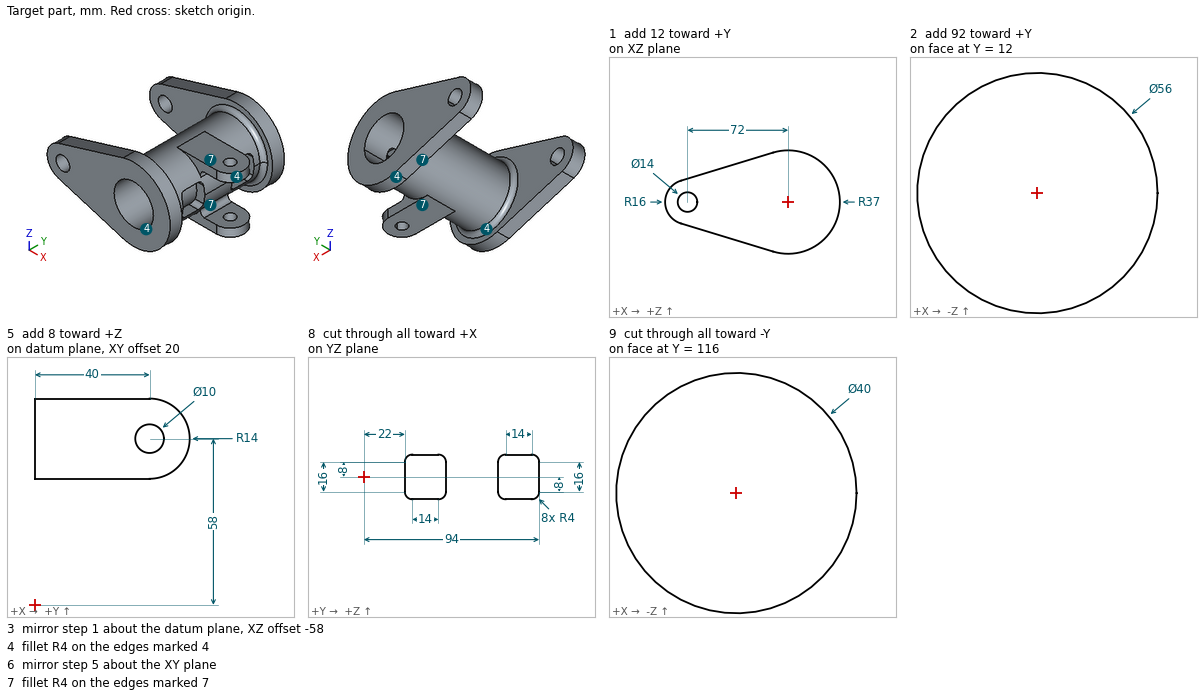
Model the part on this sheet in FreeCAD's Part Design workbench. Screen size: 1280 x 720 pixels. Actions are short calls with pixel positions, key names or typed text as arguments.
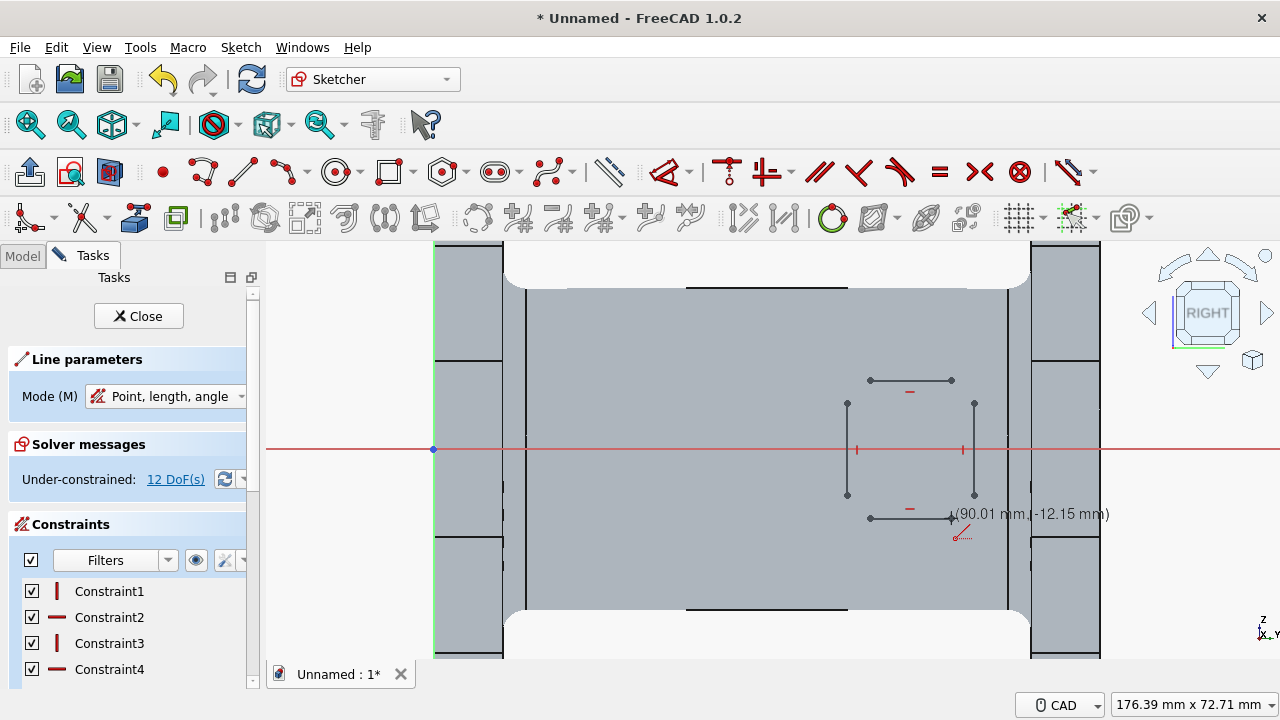
click(284, 172)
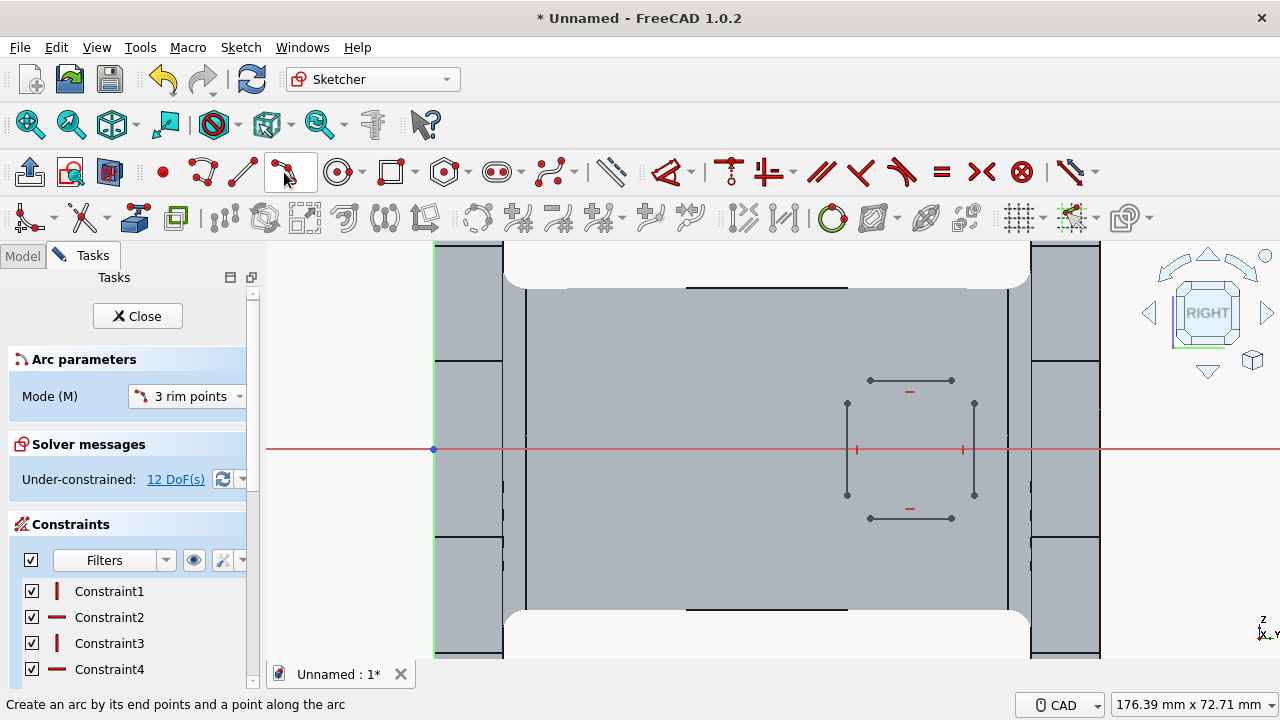
click(974, 404)
click(951, 381)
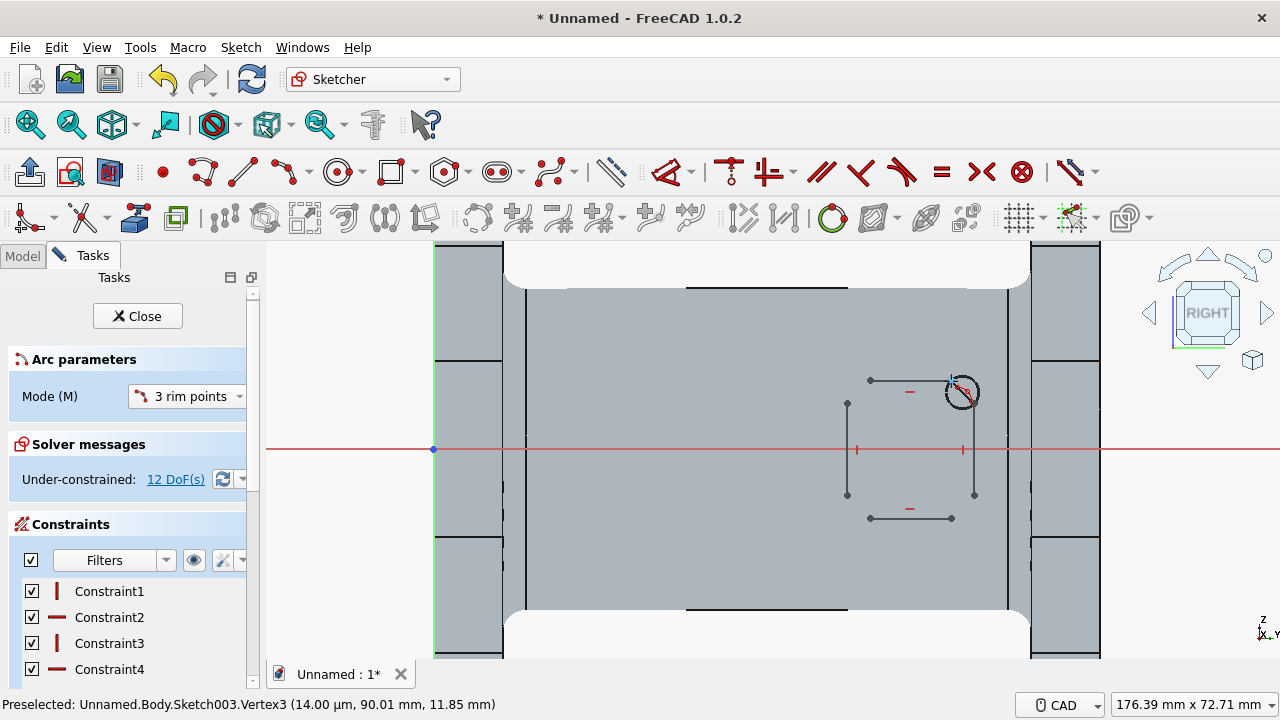
scroll(967, 387, up, 5)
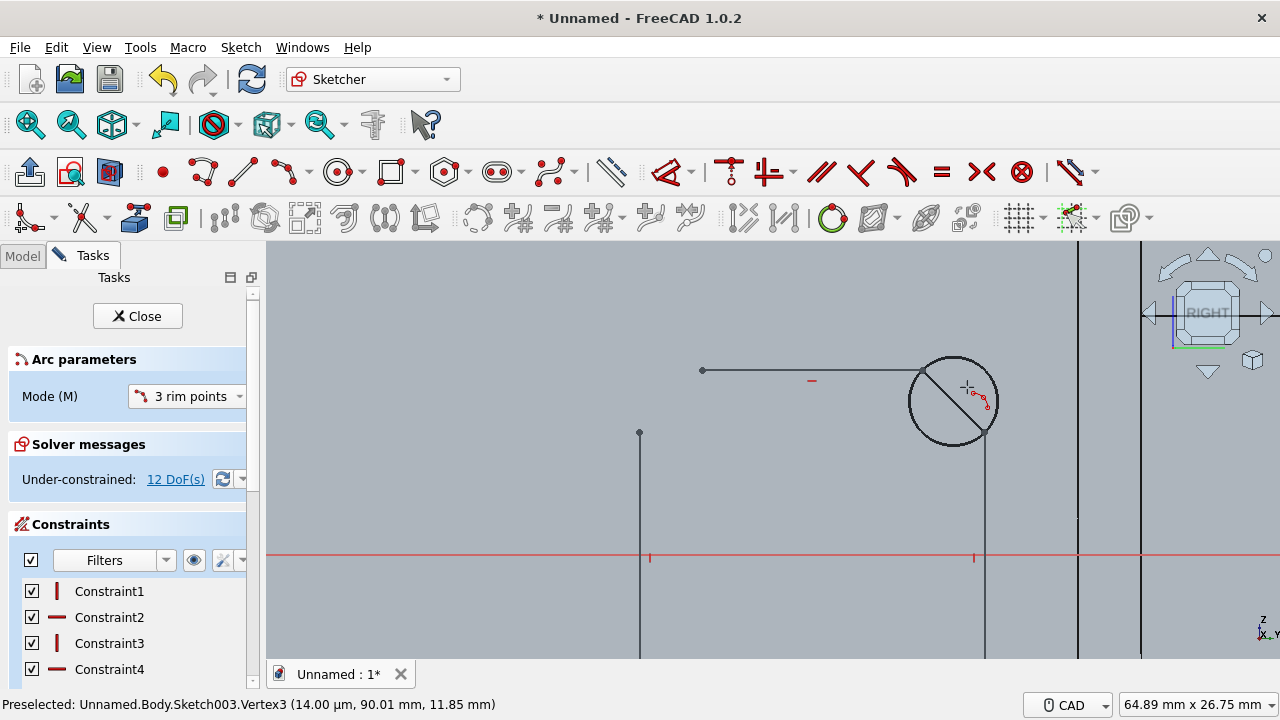
click(966, 386)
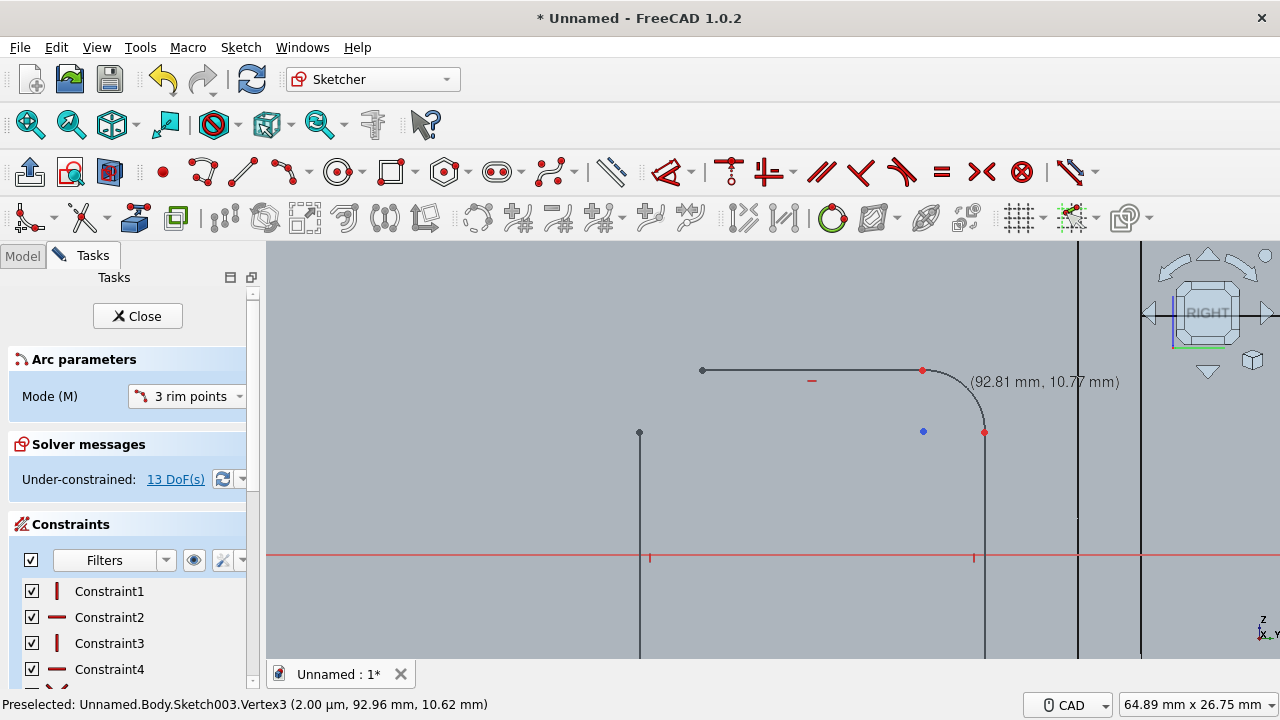
click(702, 370)
click(640, 433)
click(659, 386)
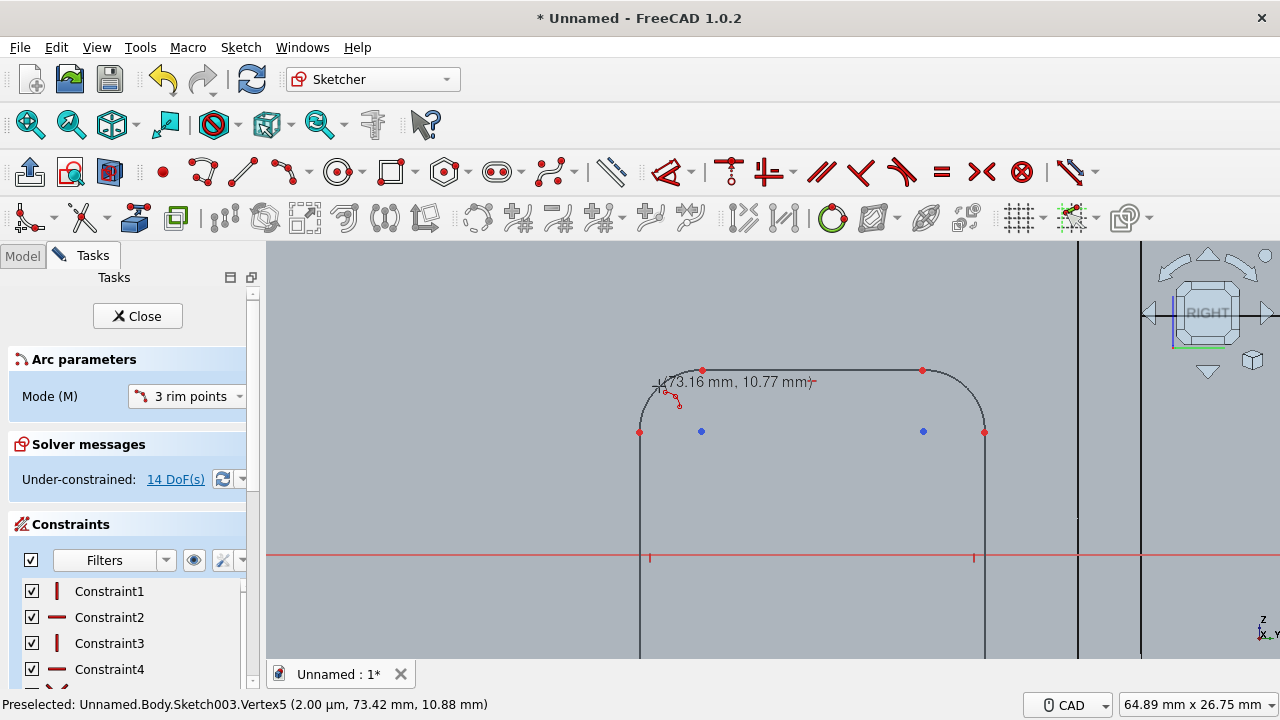
scroll(969, 389, down, 5)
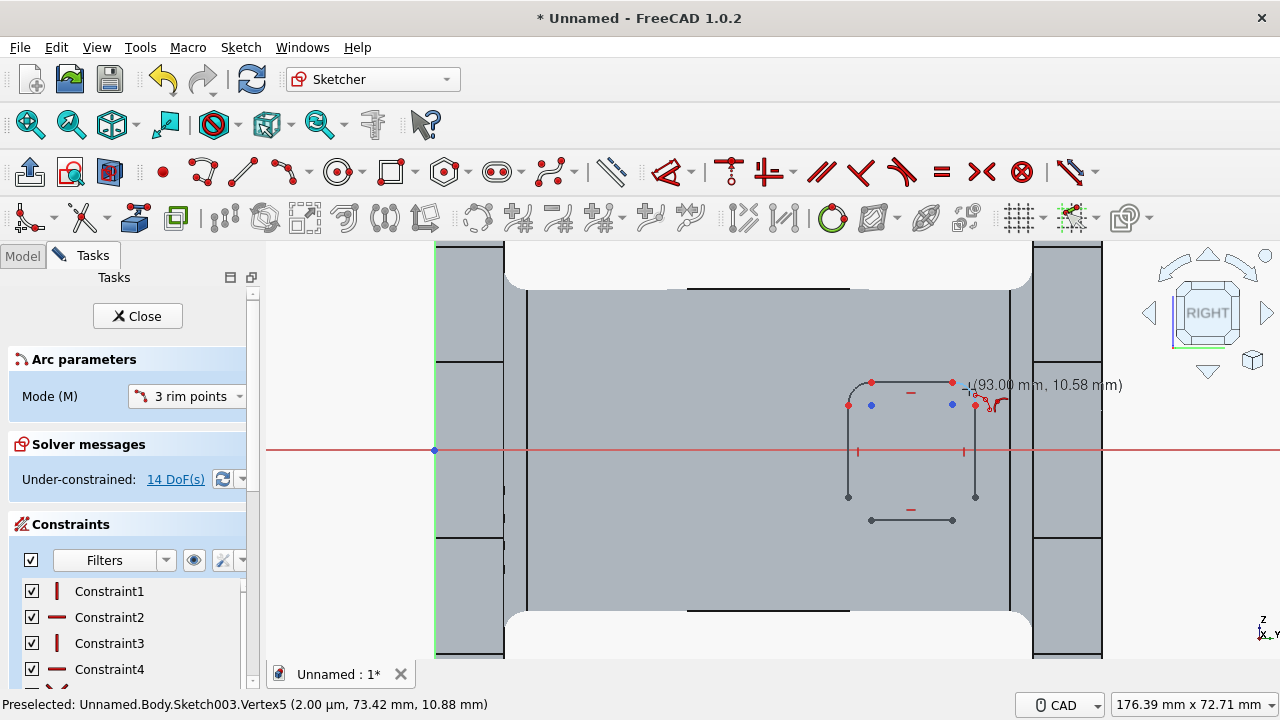
click(848, 497)
click(871, 520)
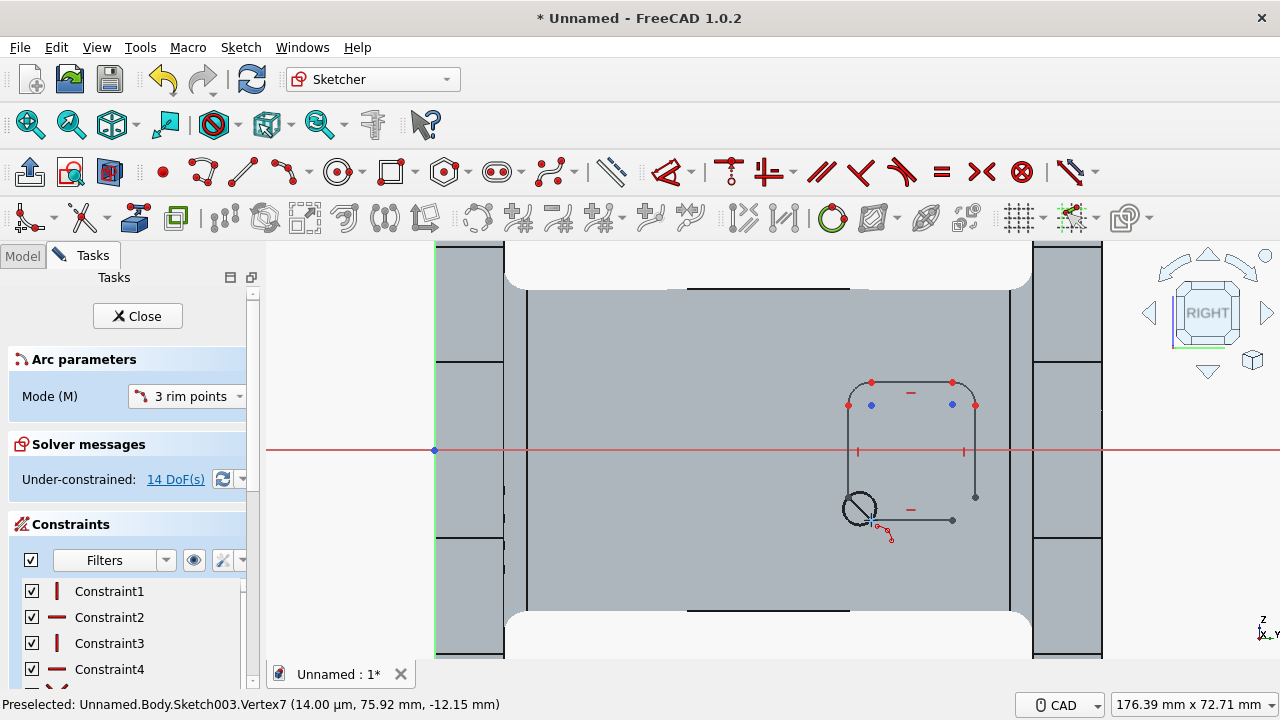
scroll(855, 513, up, 5)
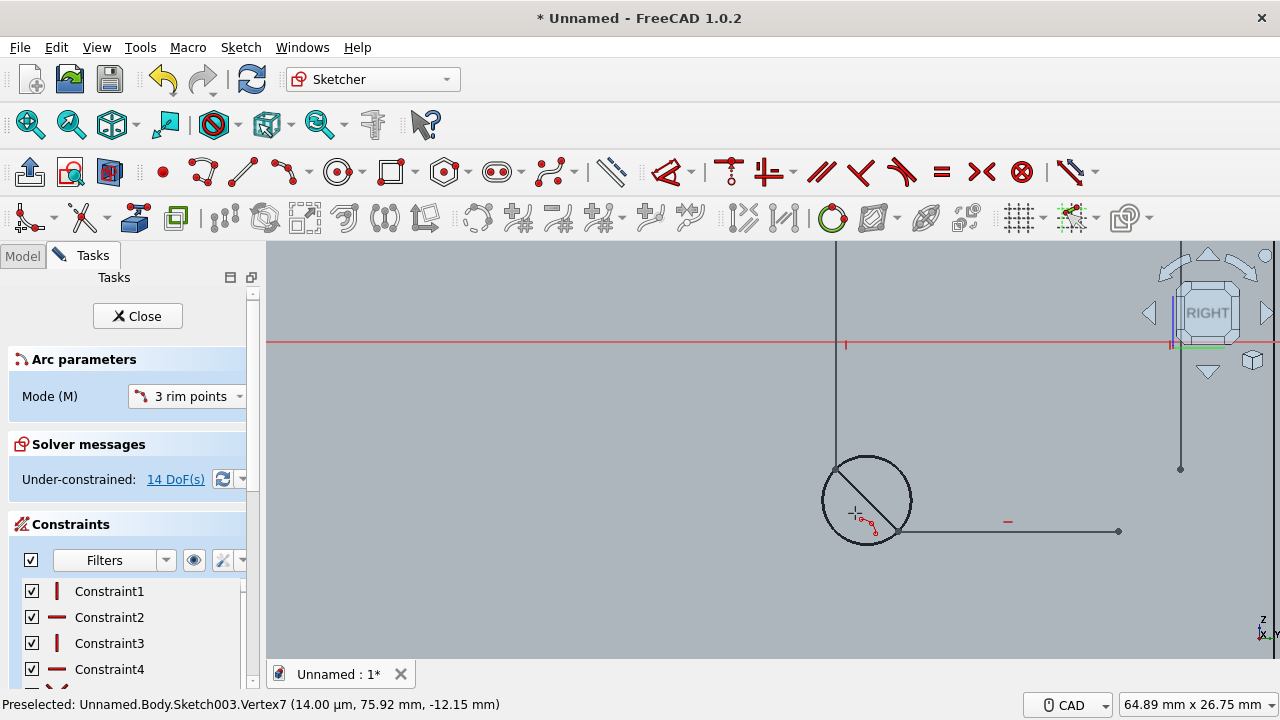
click(855, 511)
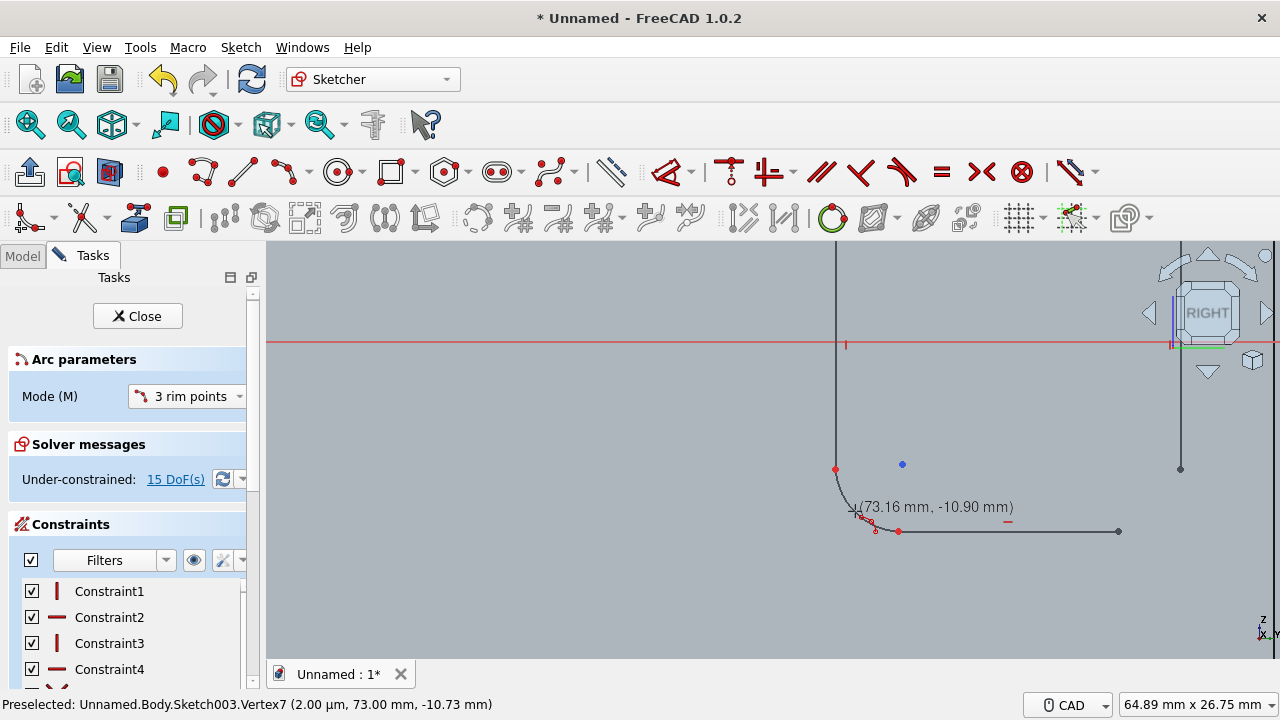
scroll(855, 513, down, 5)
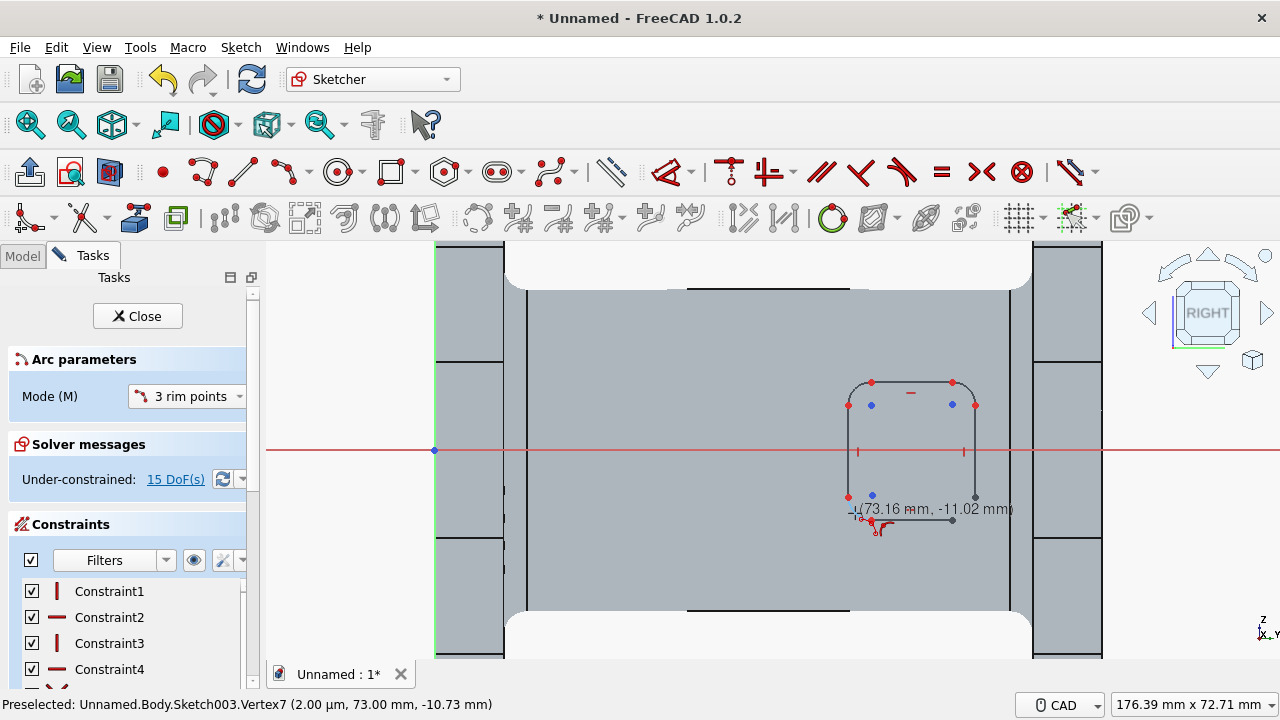
click(952, 520)
click(975, 497)